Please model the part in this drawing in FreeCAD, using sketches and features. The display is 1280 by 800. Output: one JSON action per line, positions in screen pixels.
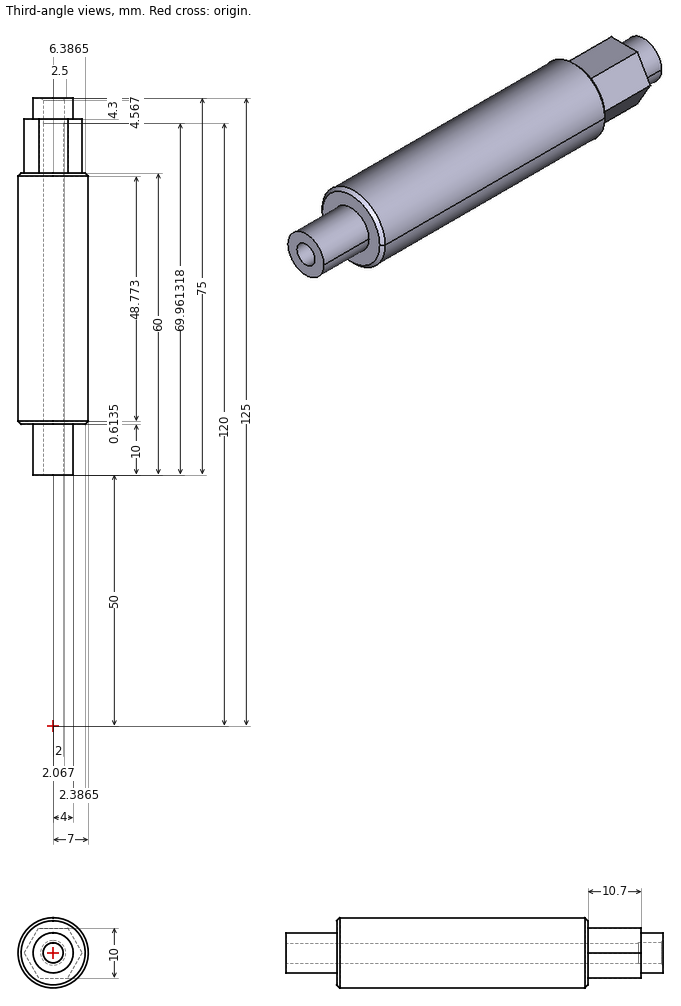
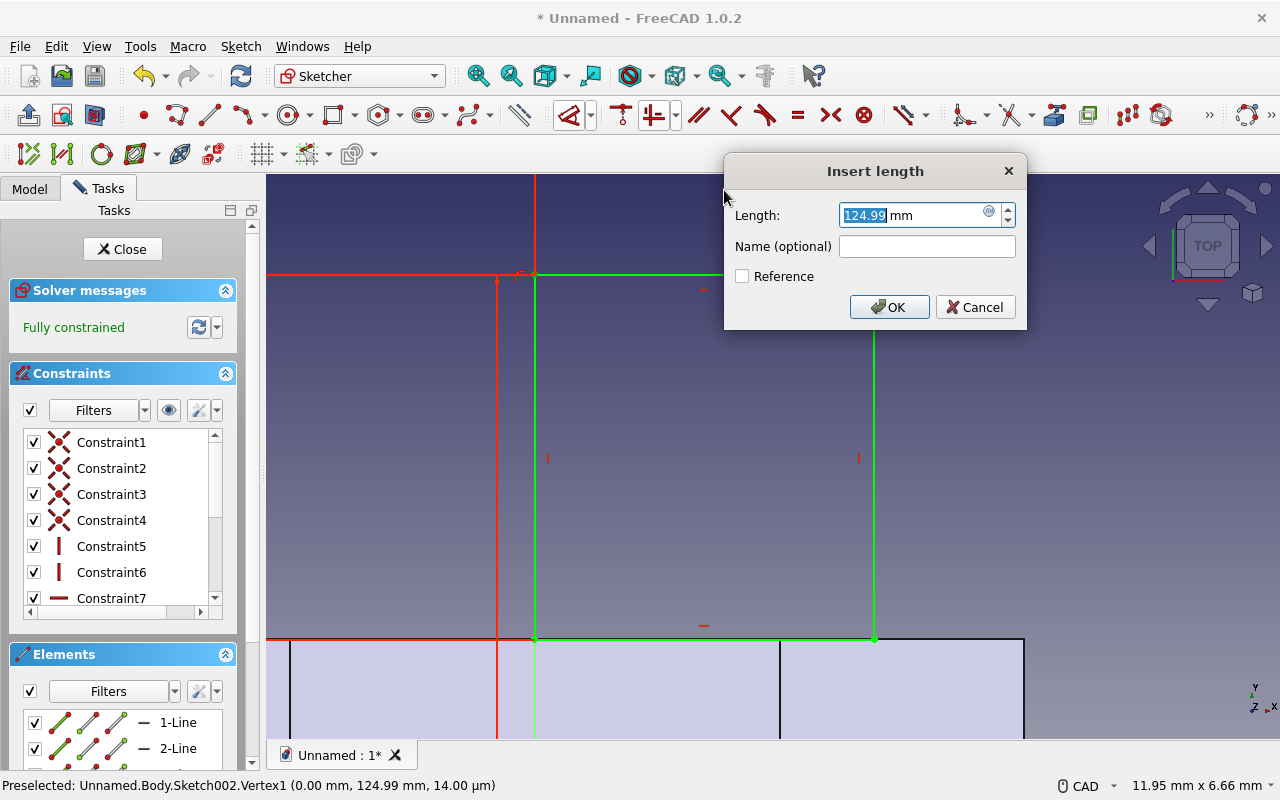
{"action": "type", "text": "125"}
{"action": "key", "text": "Return"}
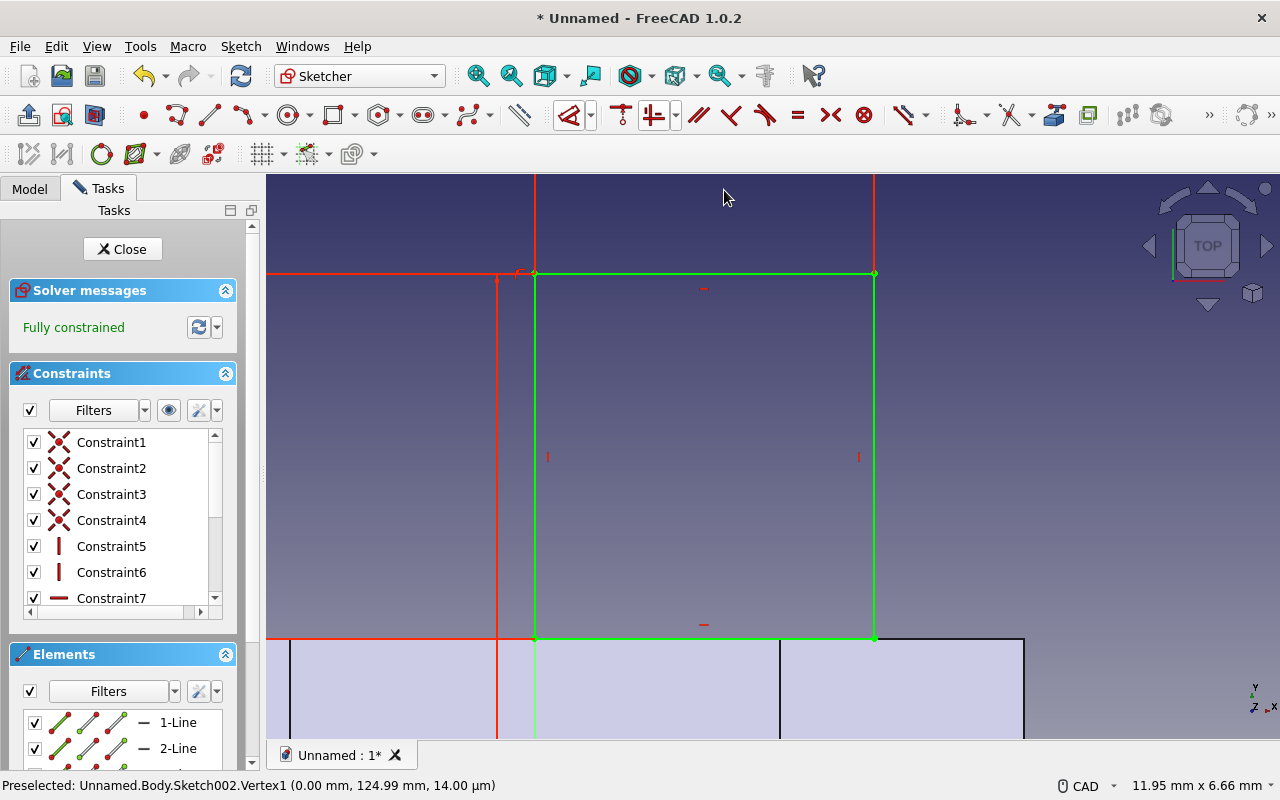
{"action": "left_click", "coordinate": [123, 249]}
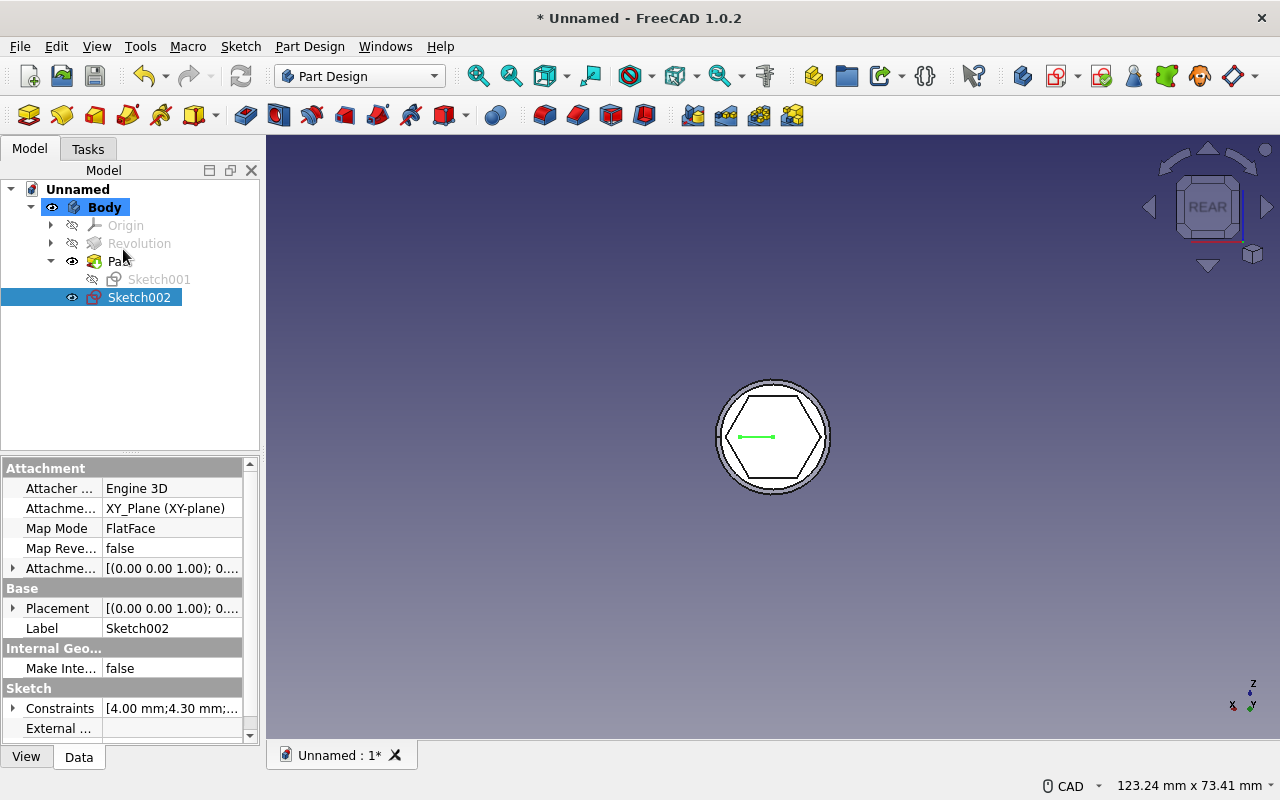
{"action": "left_click", "coordinate": [62, 116]}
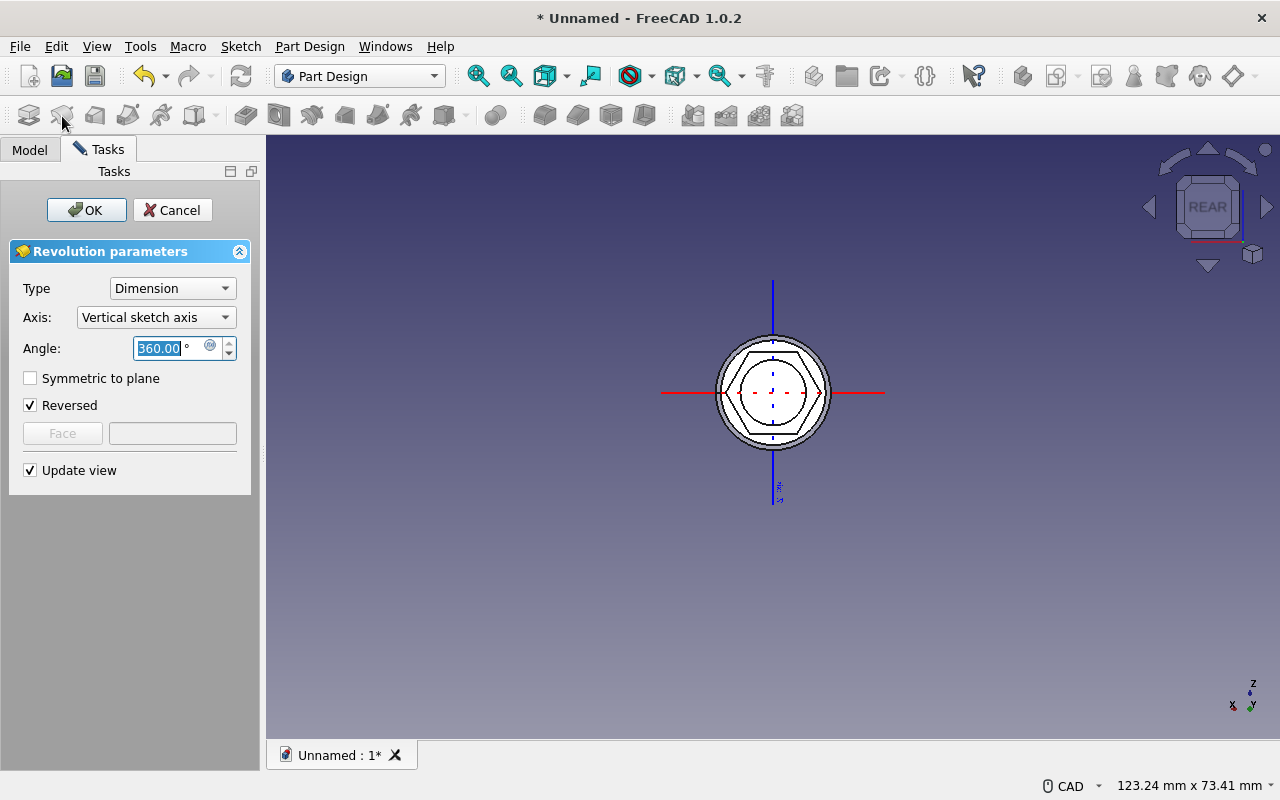
{"action": "left_click", "coordinate": [87, 210]}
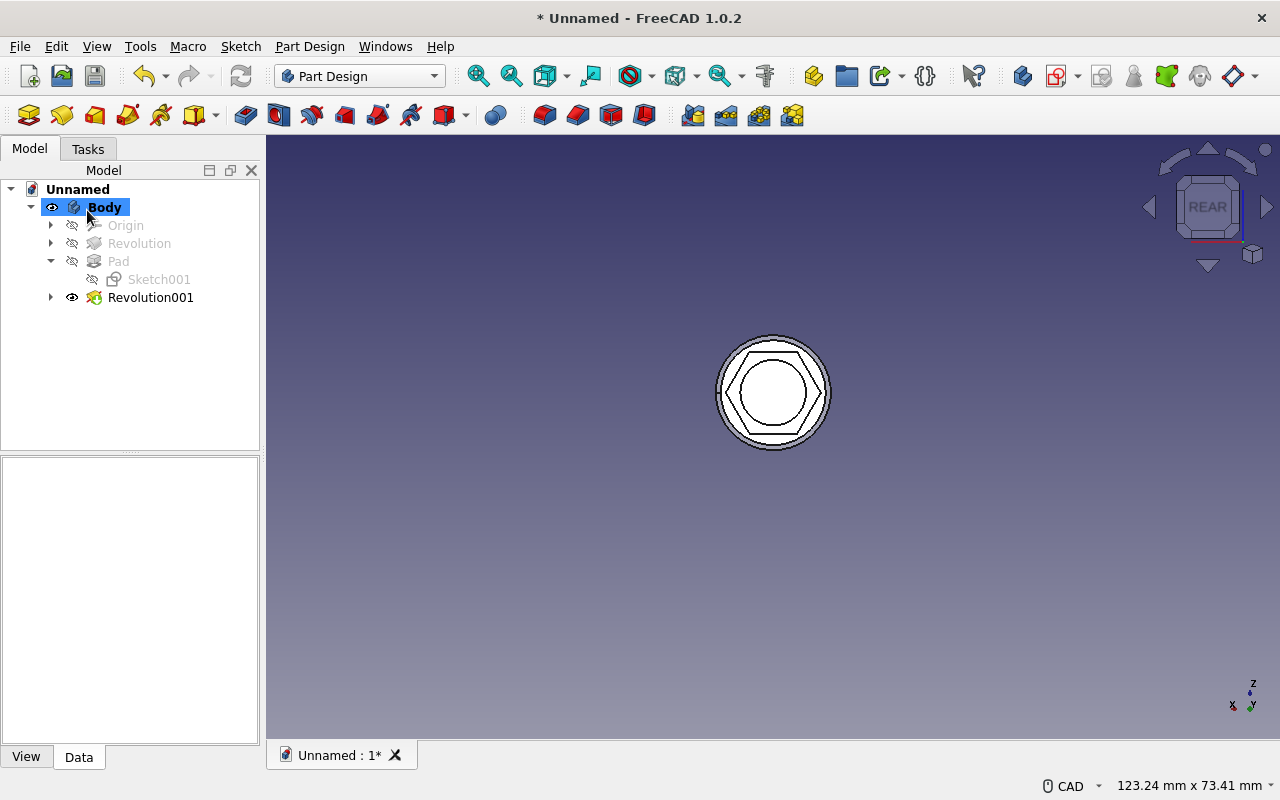
{"action": "key", "text": "v f"}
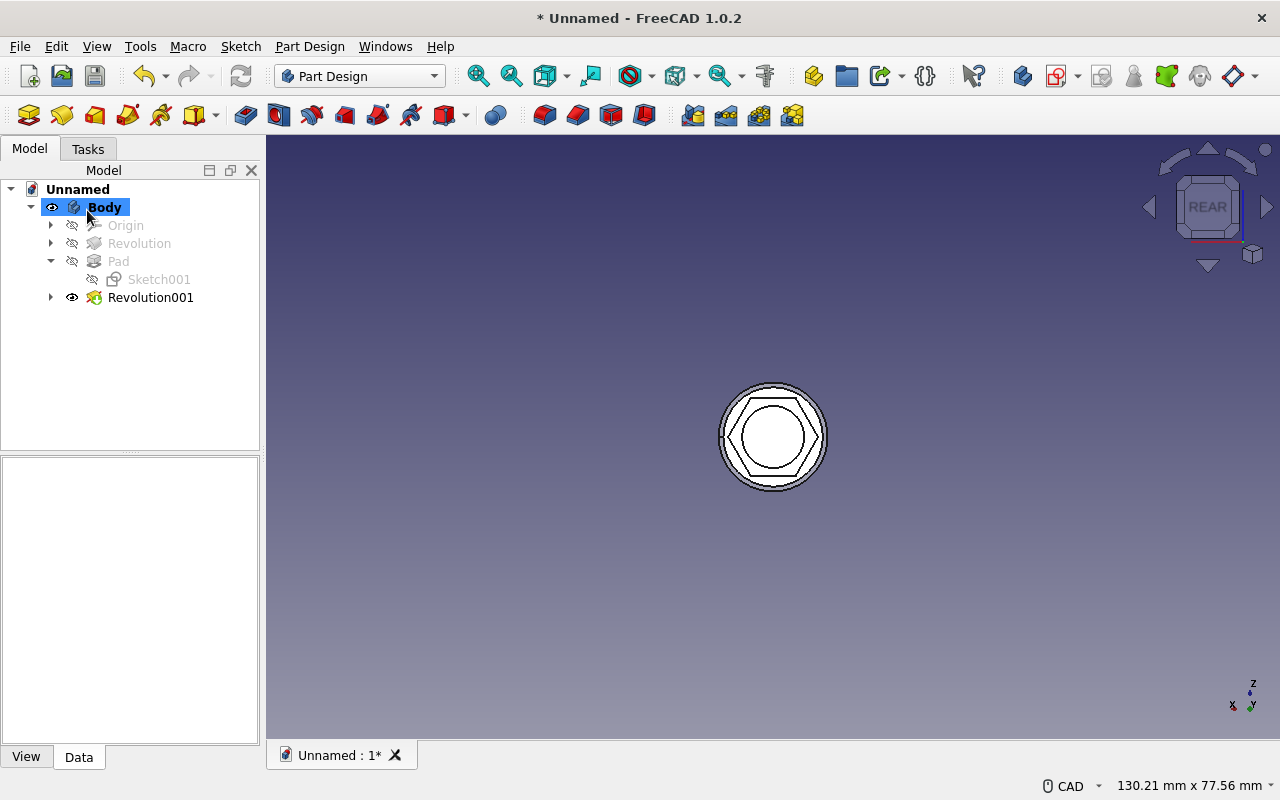
{"action": "left_click", "coordinate": [1056, 76]}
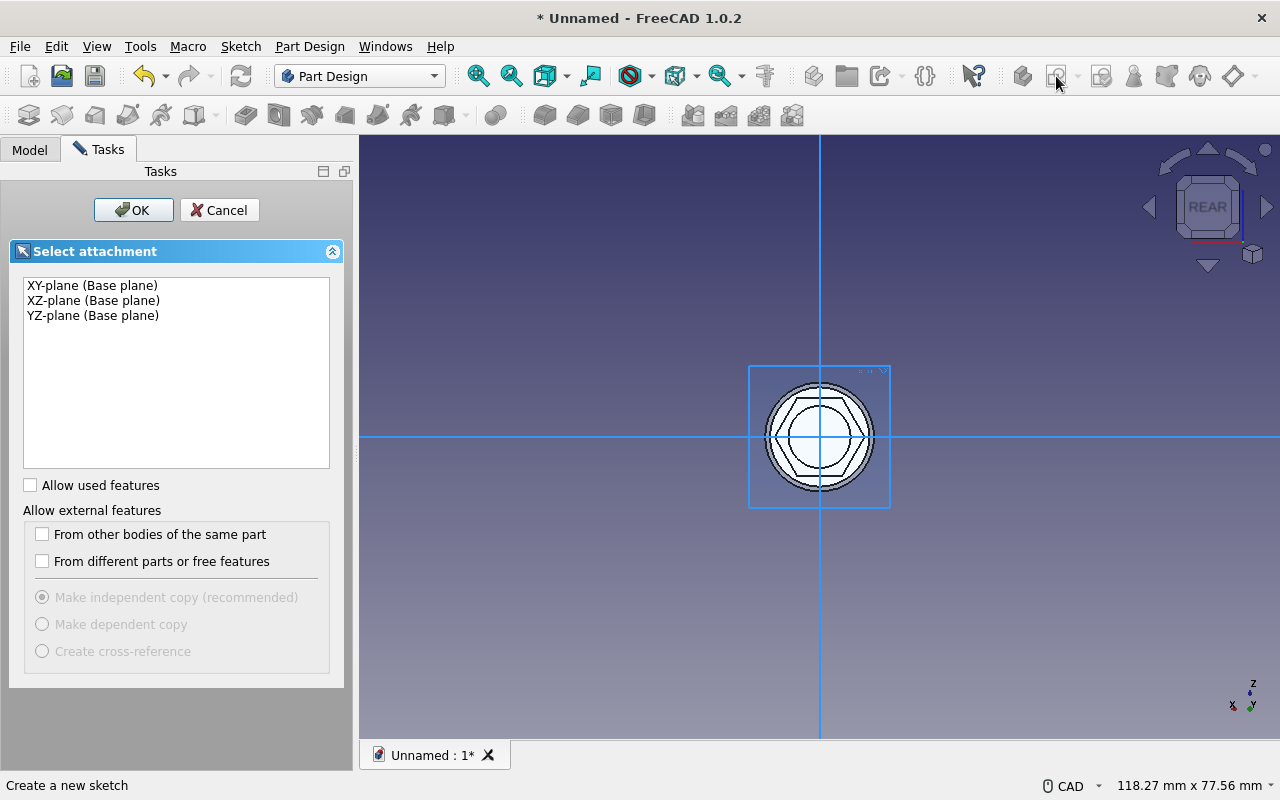
{"action": "left_click", "coordinate": [84, 286]}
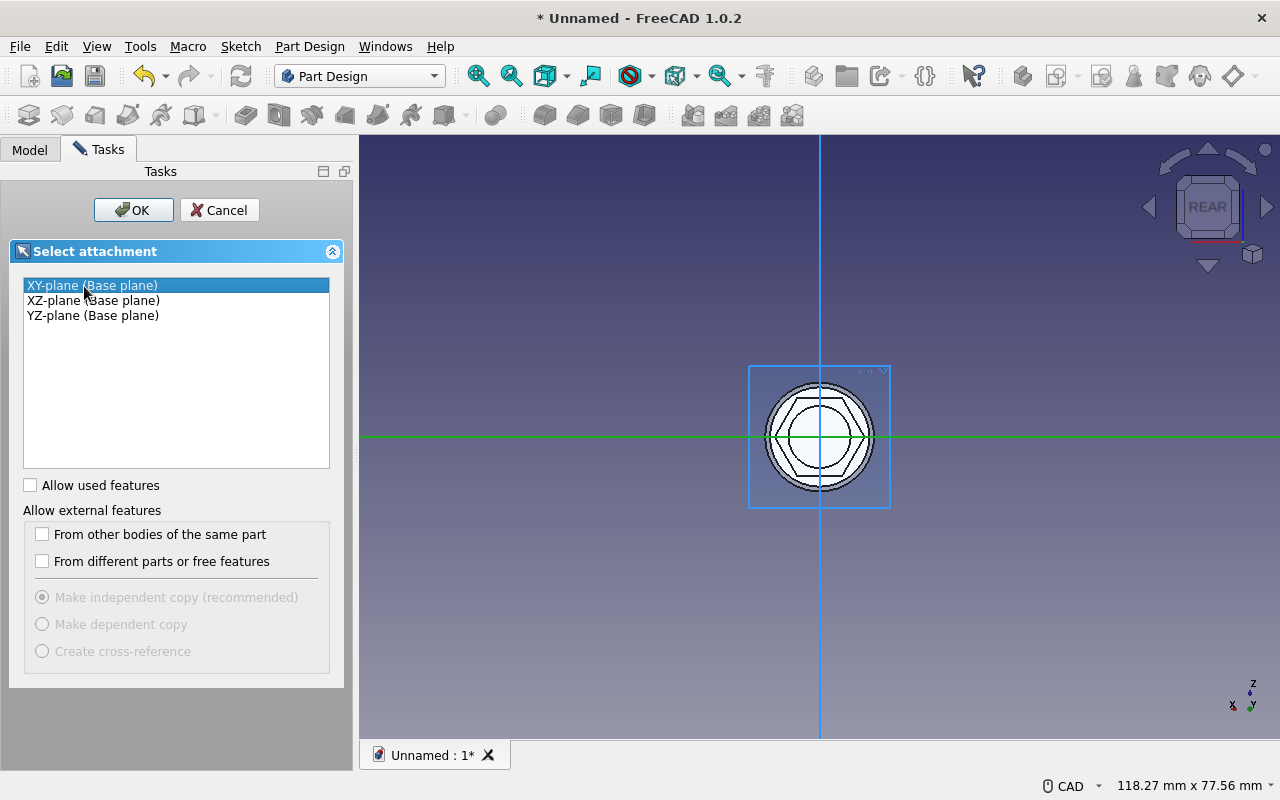
{"action": "left_click", "coordinate": [134, 210]}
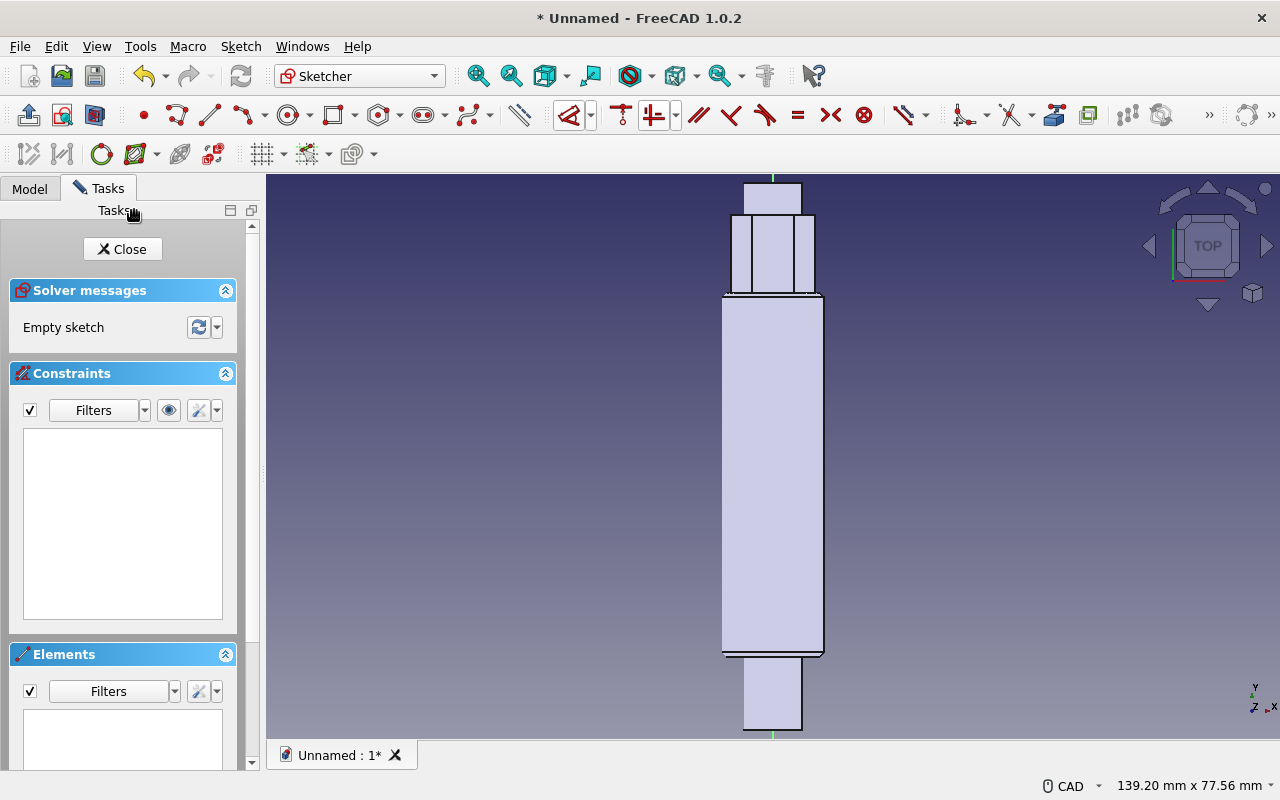
{"action": "left_click", "coordinate": [95, 116]}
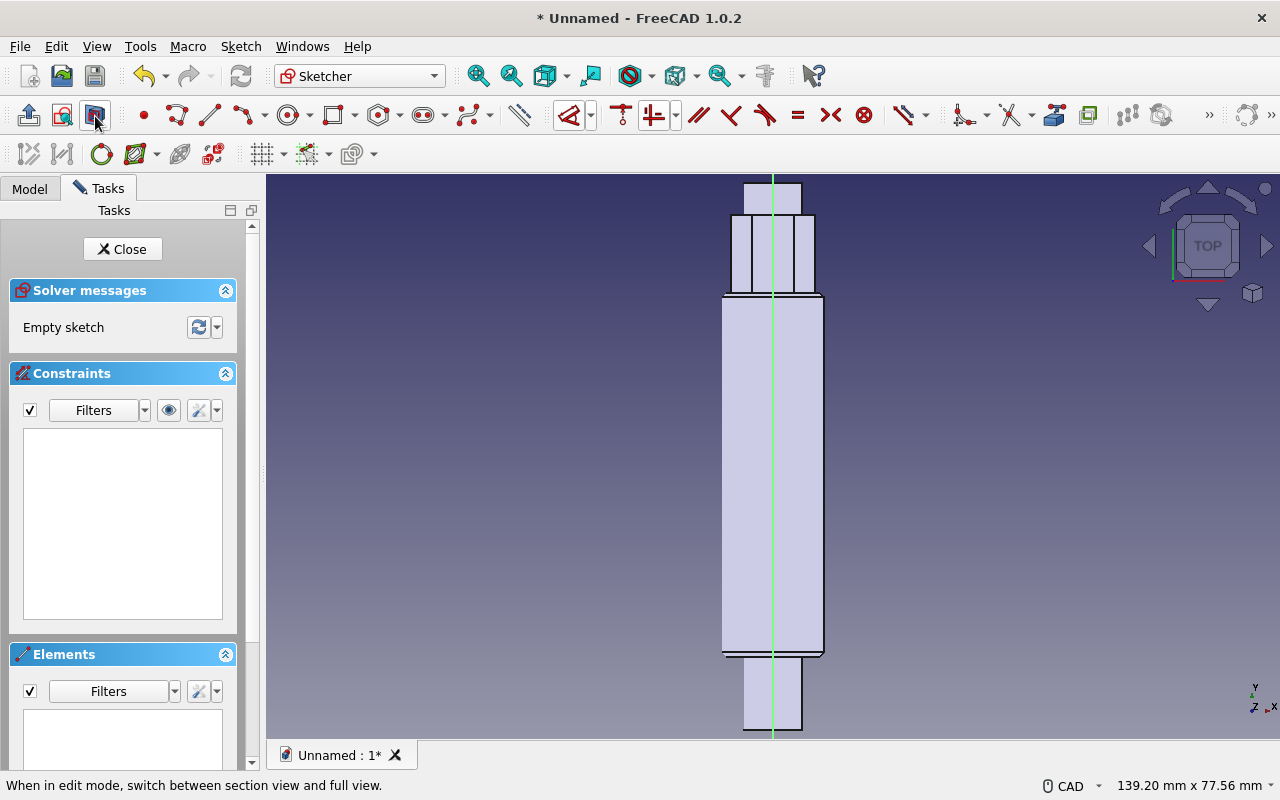
{"action": "scroll", "coordinate": [659, 351], "scroll_direction": "down", "scroll_amount": 5}